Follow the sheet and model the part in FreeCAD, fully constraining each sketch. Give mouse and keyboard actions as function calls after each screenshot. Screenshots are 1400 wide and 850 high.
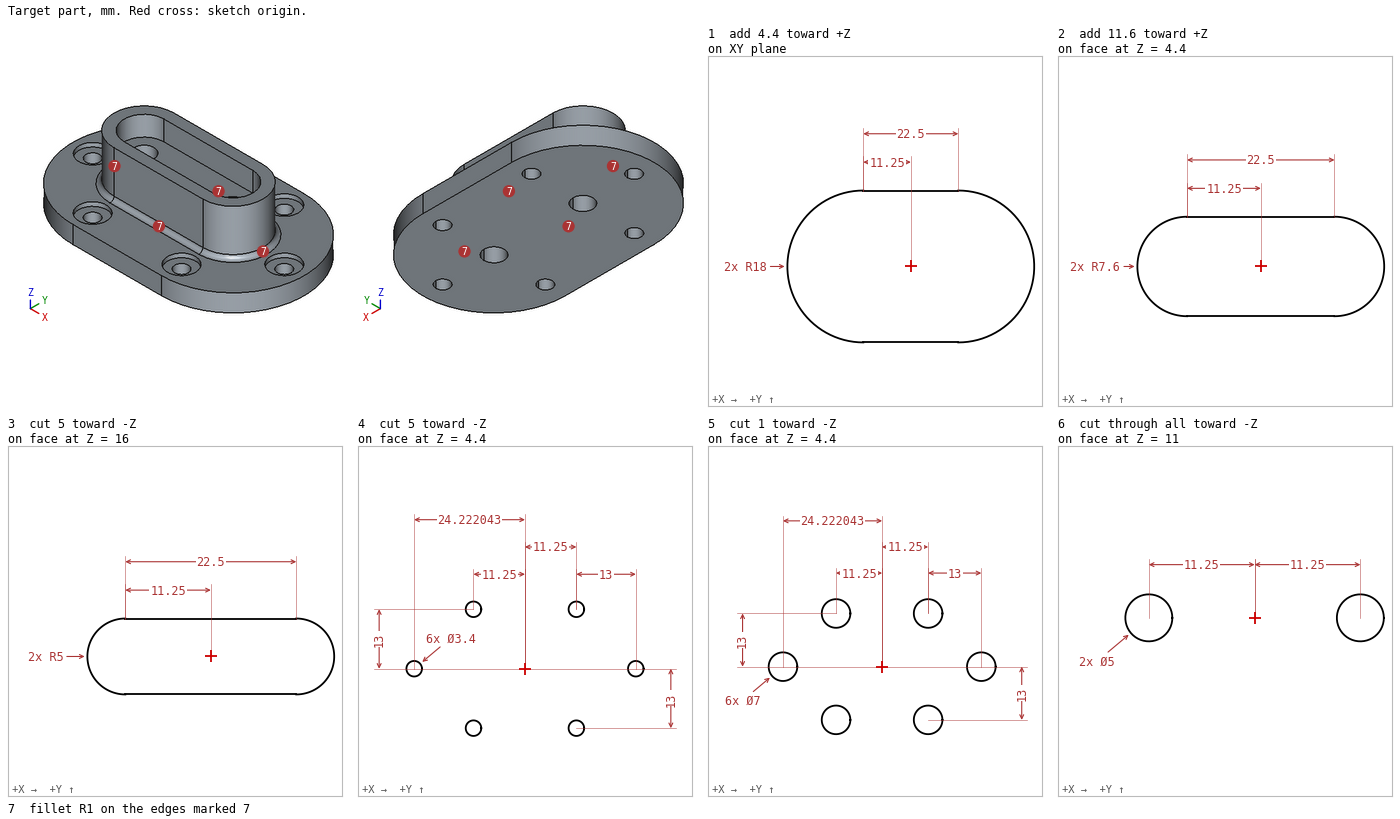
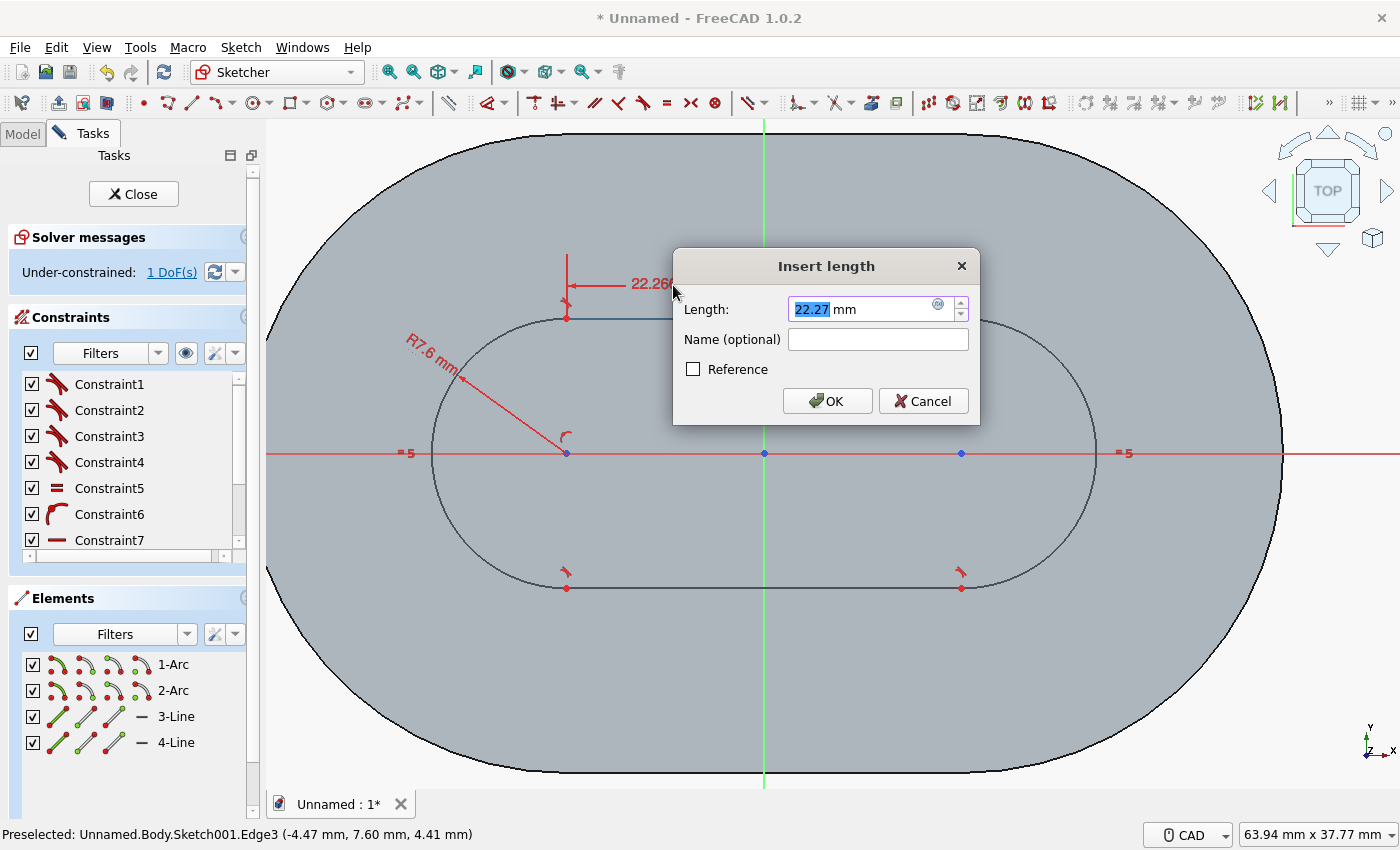
text(22.5)
key(Return)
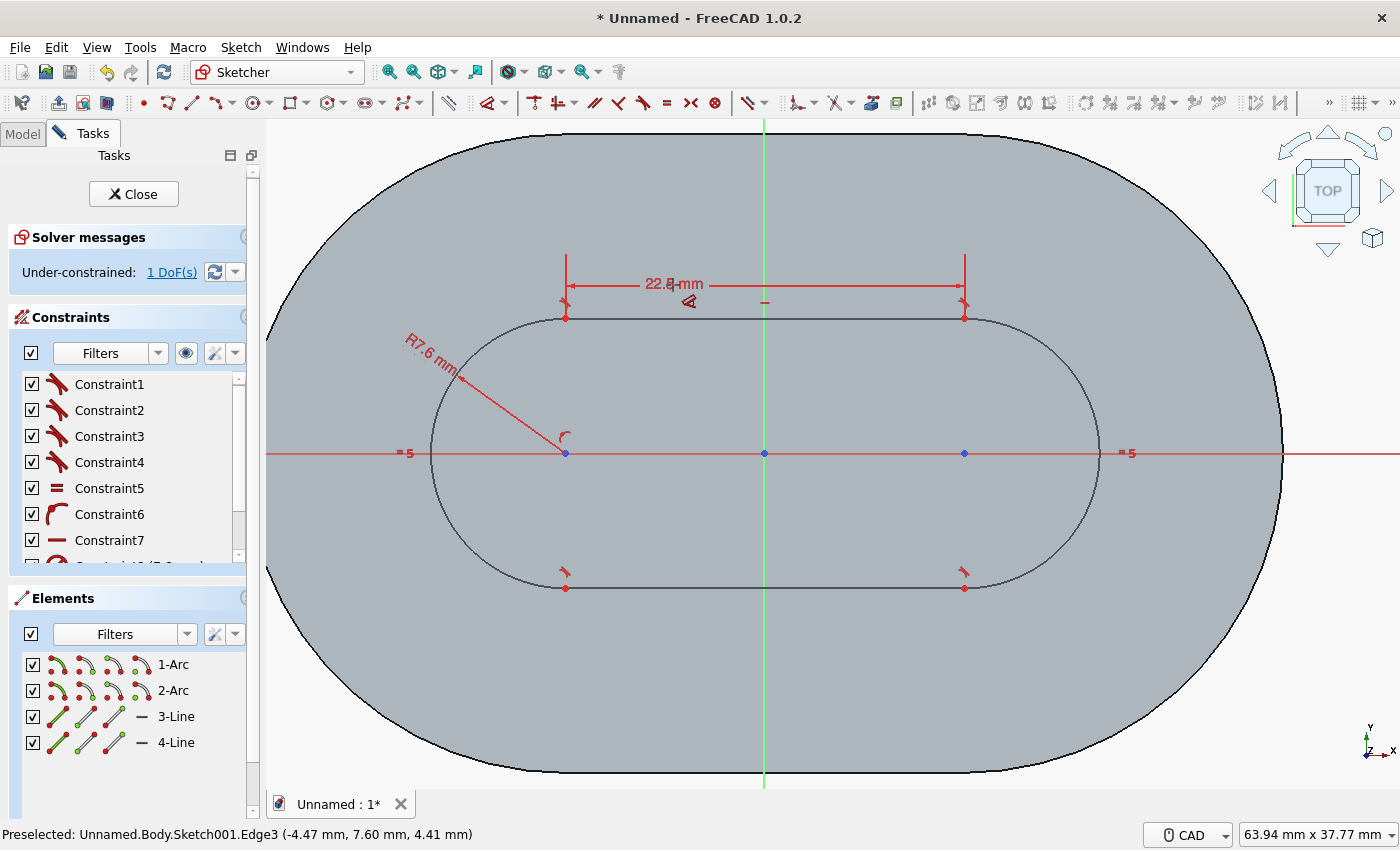
click(566, 319)
click(596, 285)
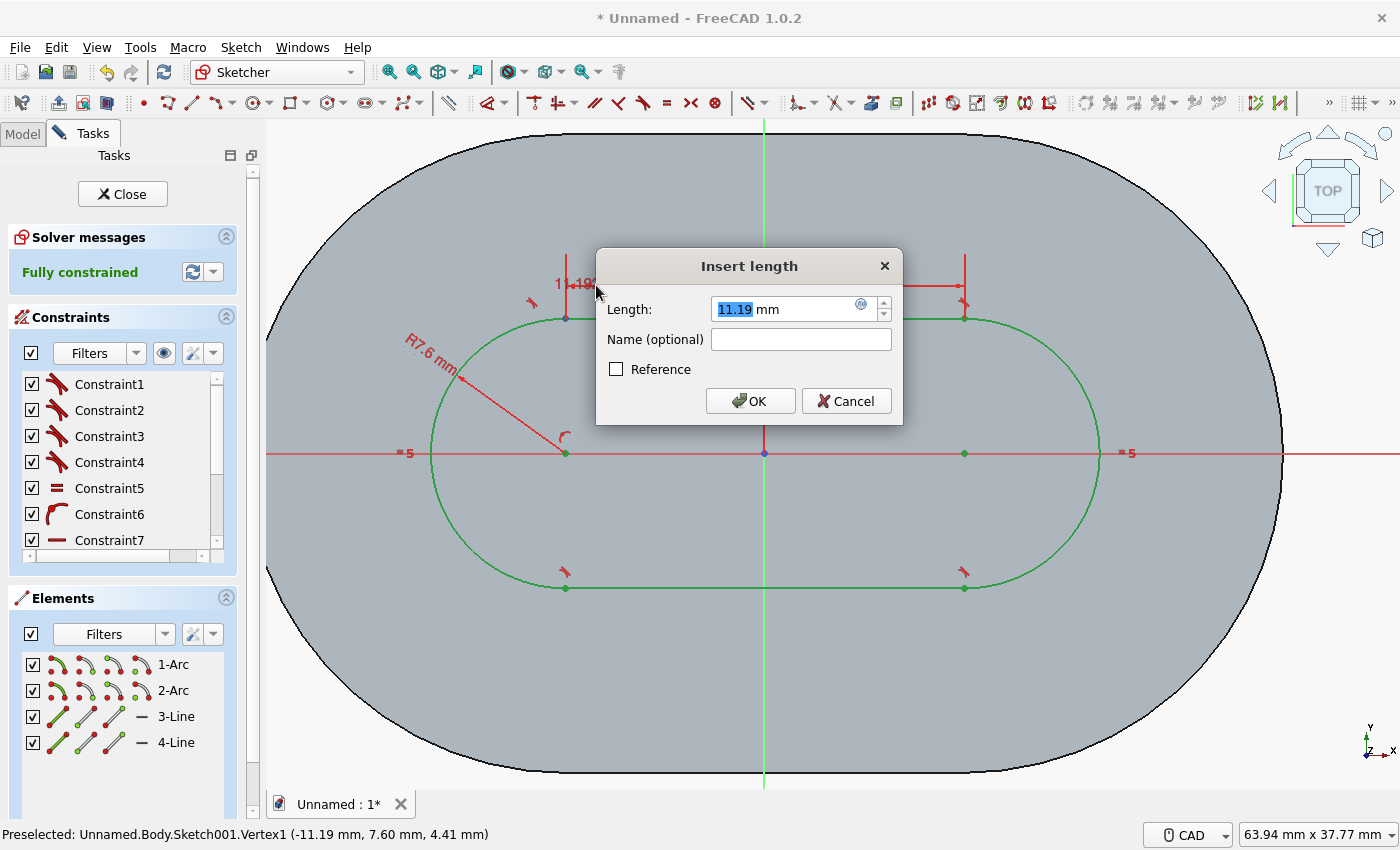
text(11.25)
key(Return)
key(Escape)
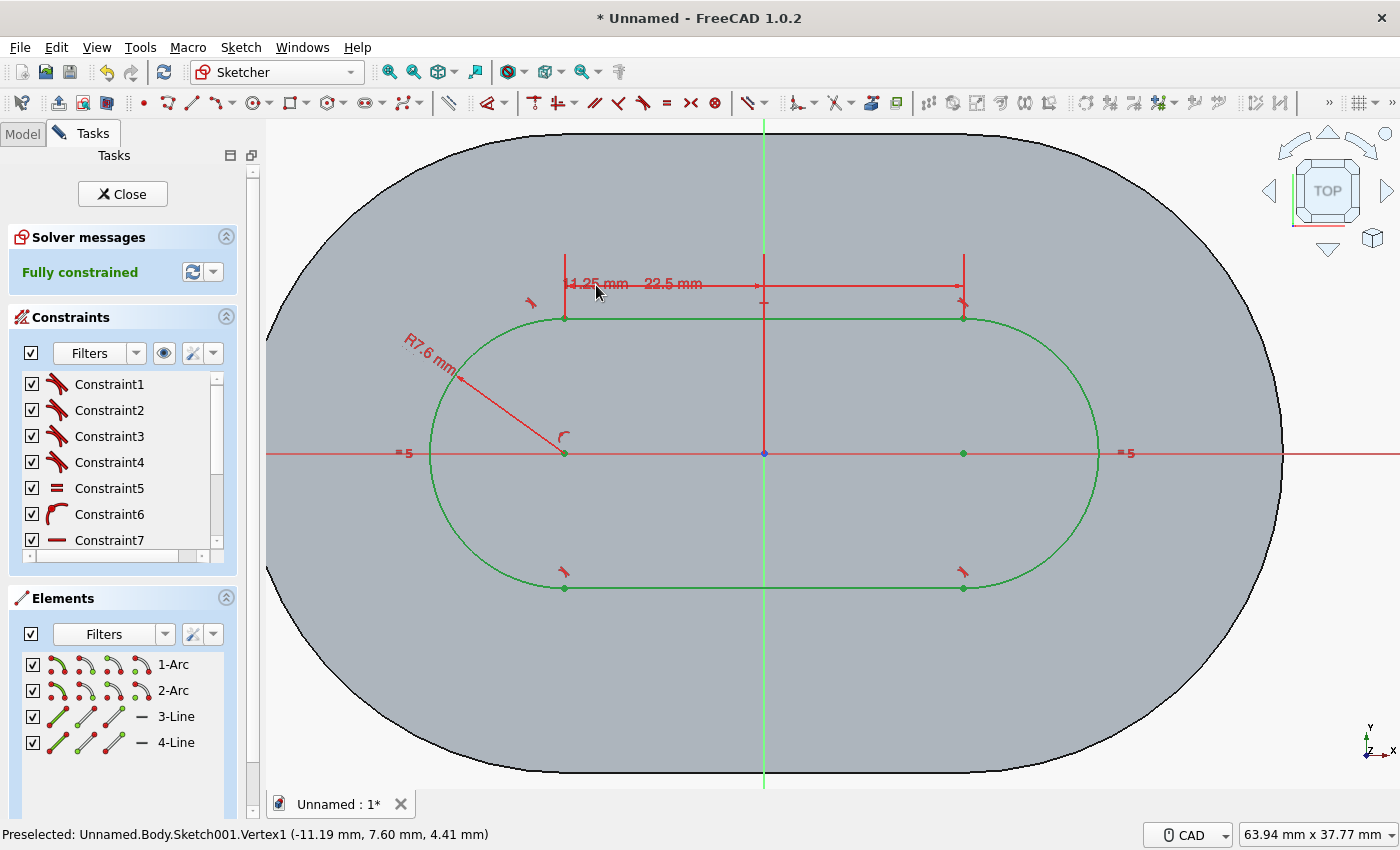
click(123, 194)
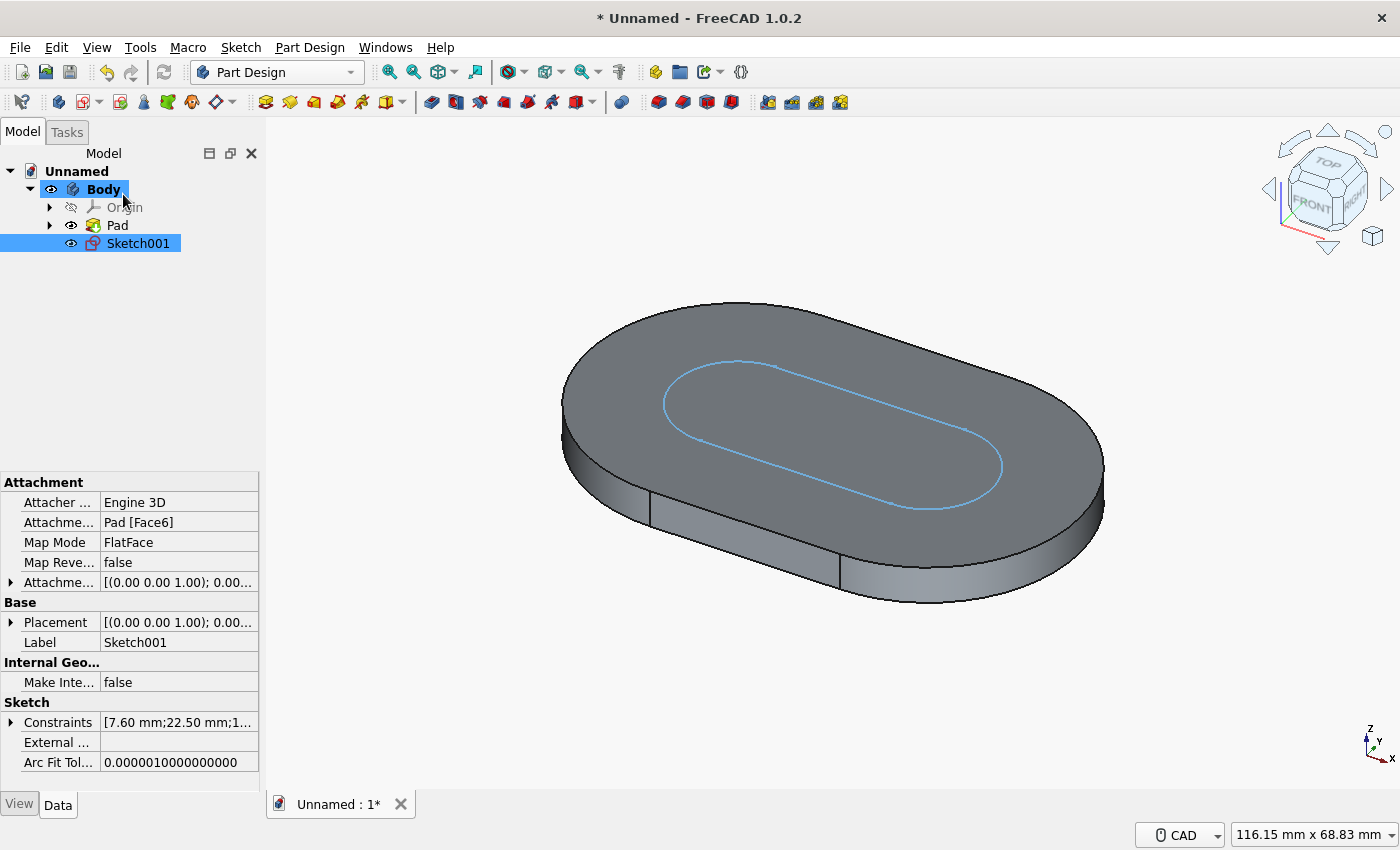
click(266, 102)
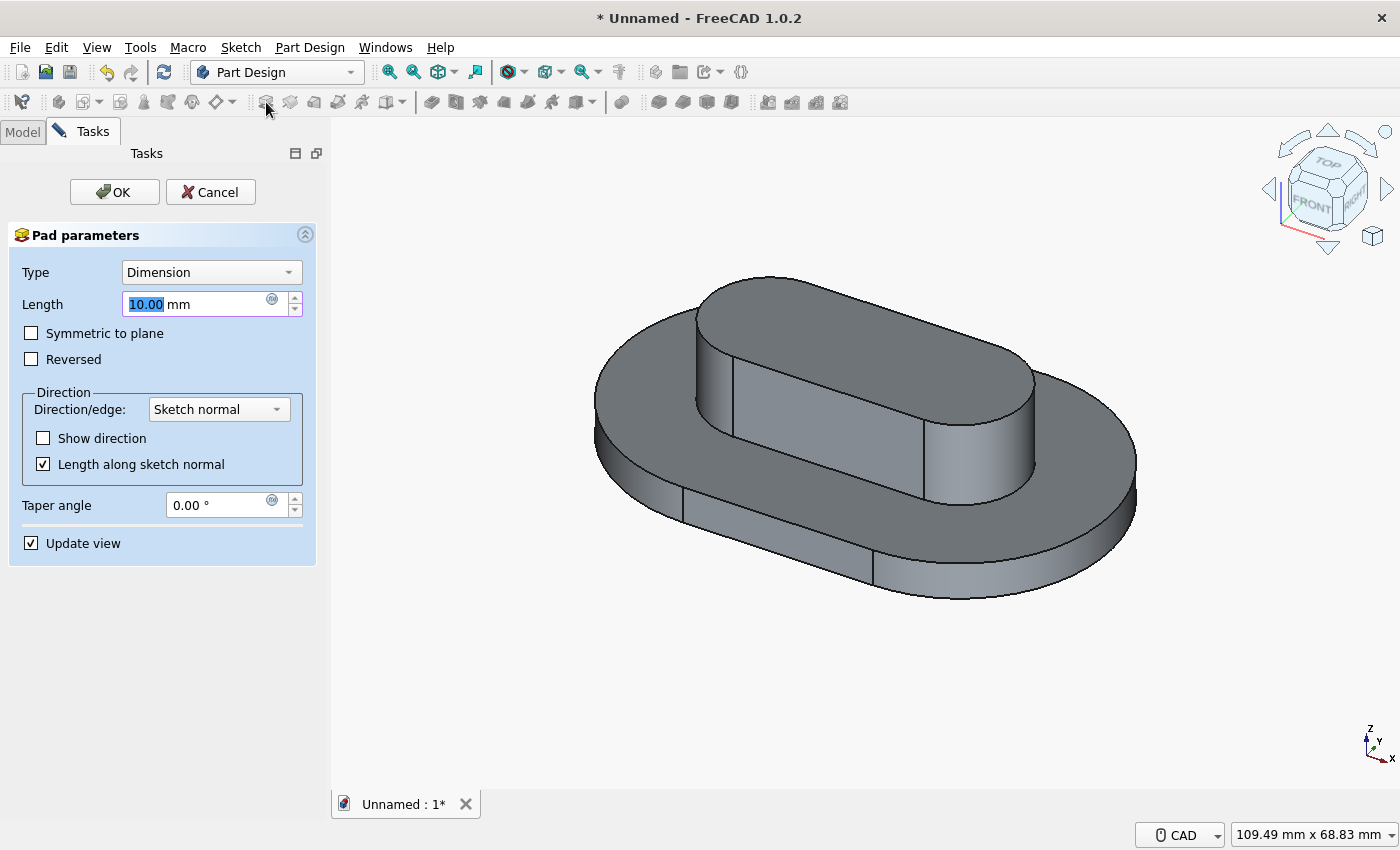
text(11.6)
key(Tab)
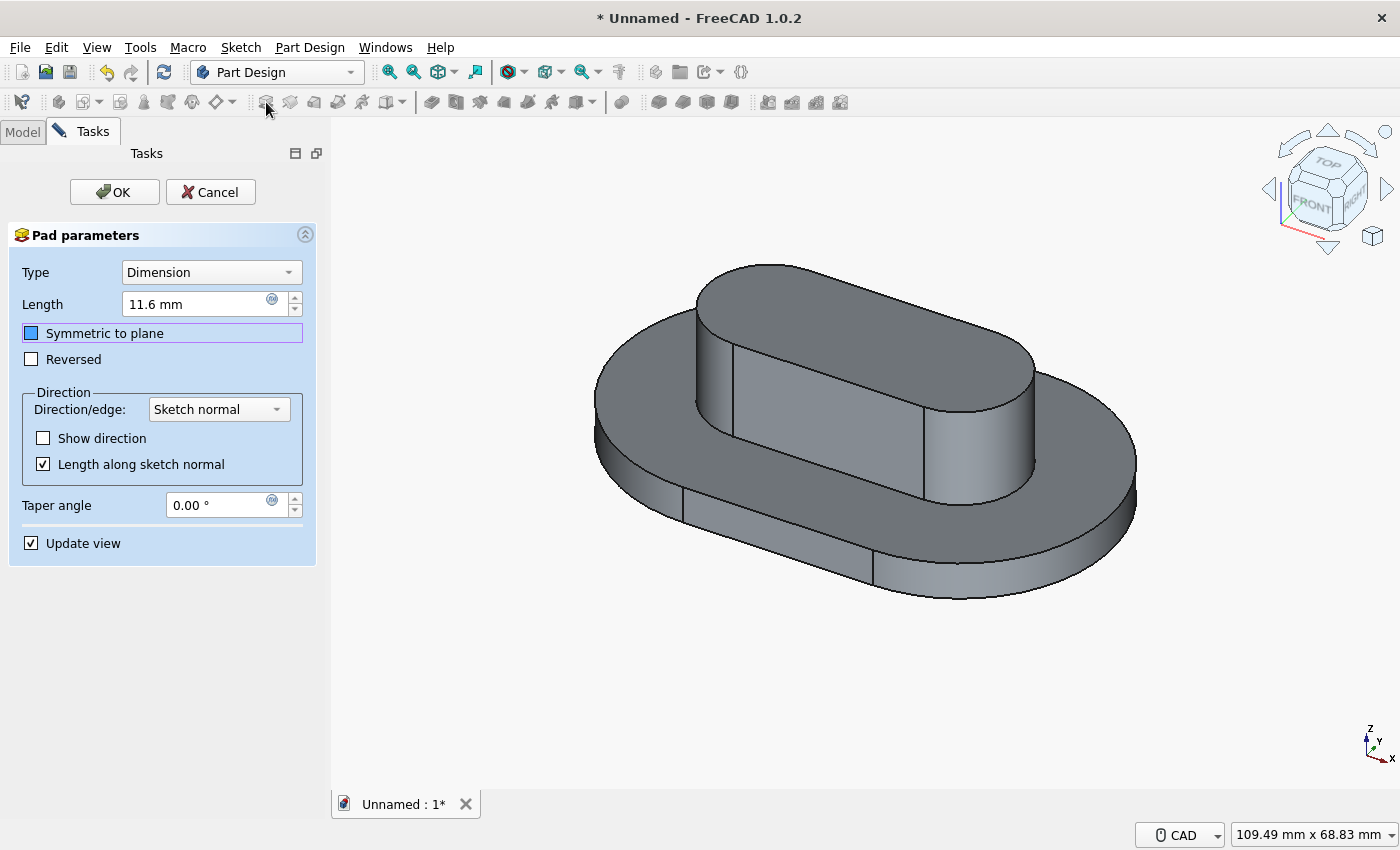
click(115, 192)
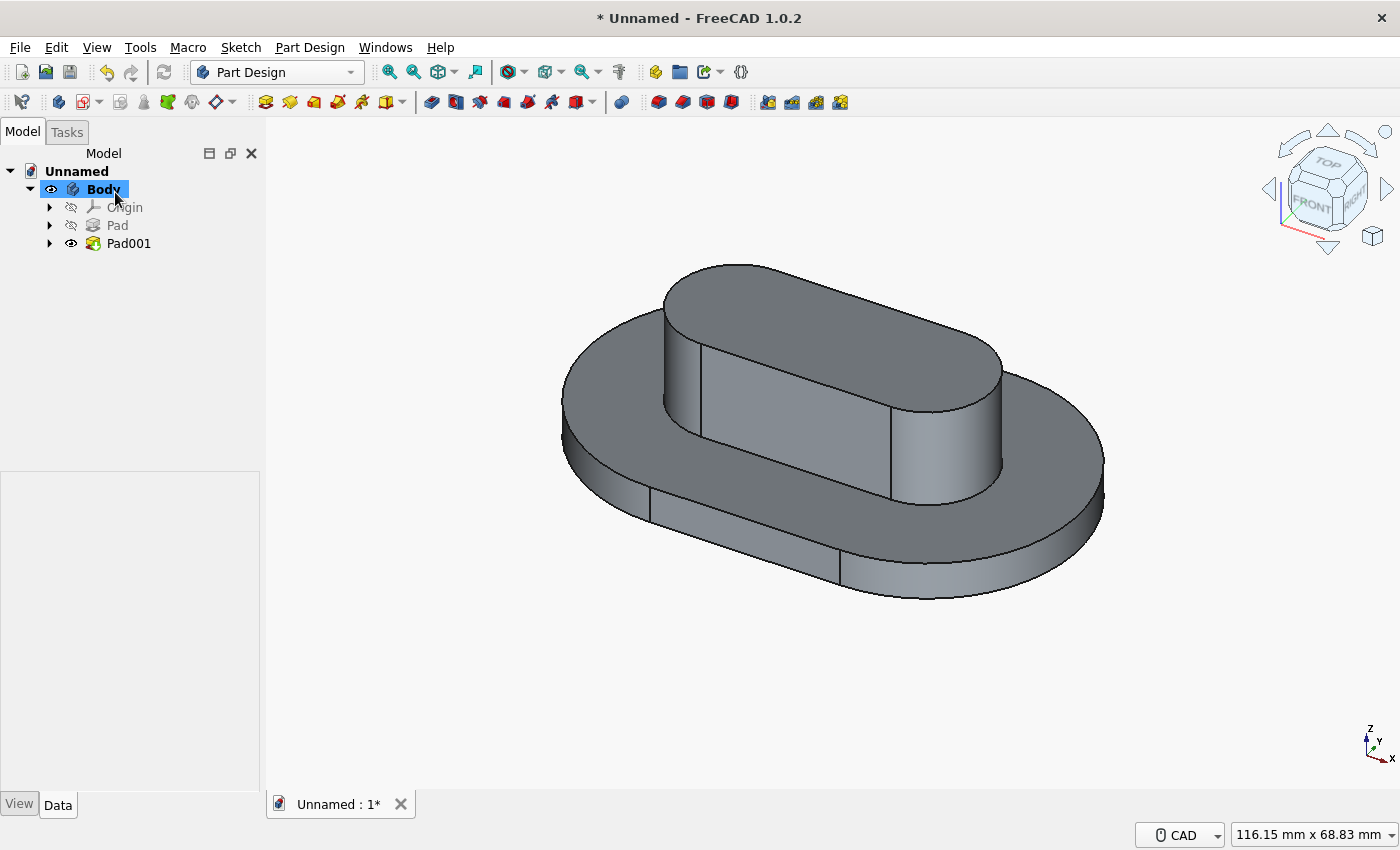
click(924, 368)